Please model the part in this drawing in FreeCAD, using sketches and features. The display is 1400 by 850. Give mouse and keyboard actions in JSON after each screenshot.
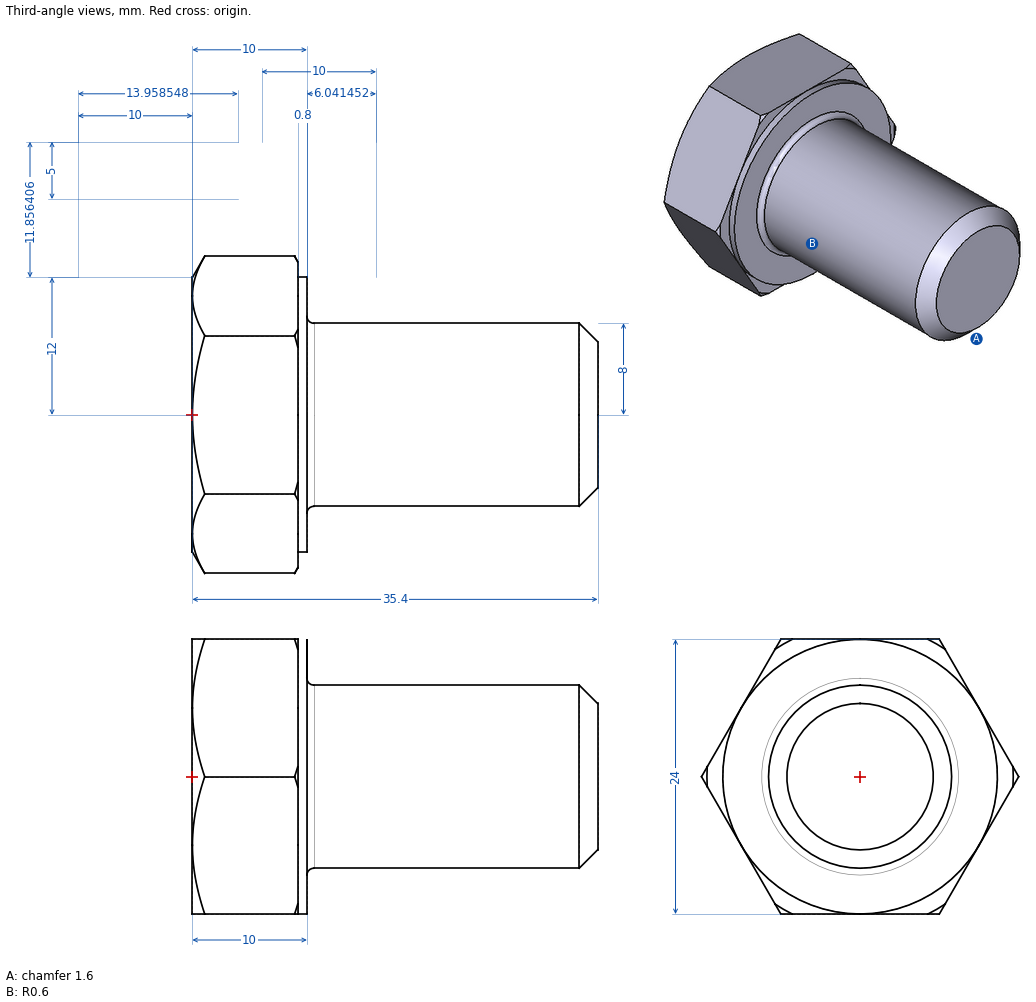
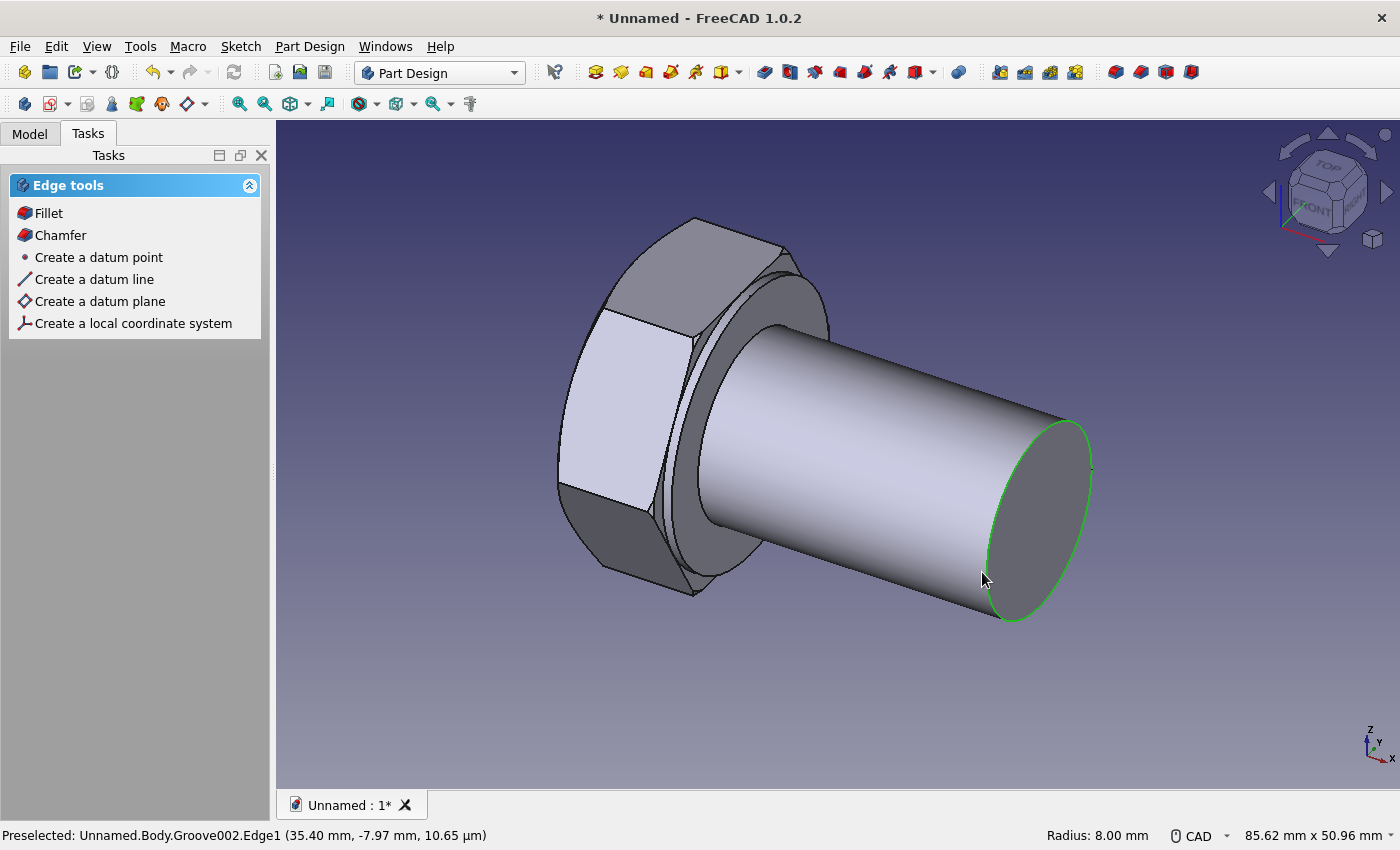
{"action": "left_click", "coordinate": [1141, 72]}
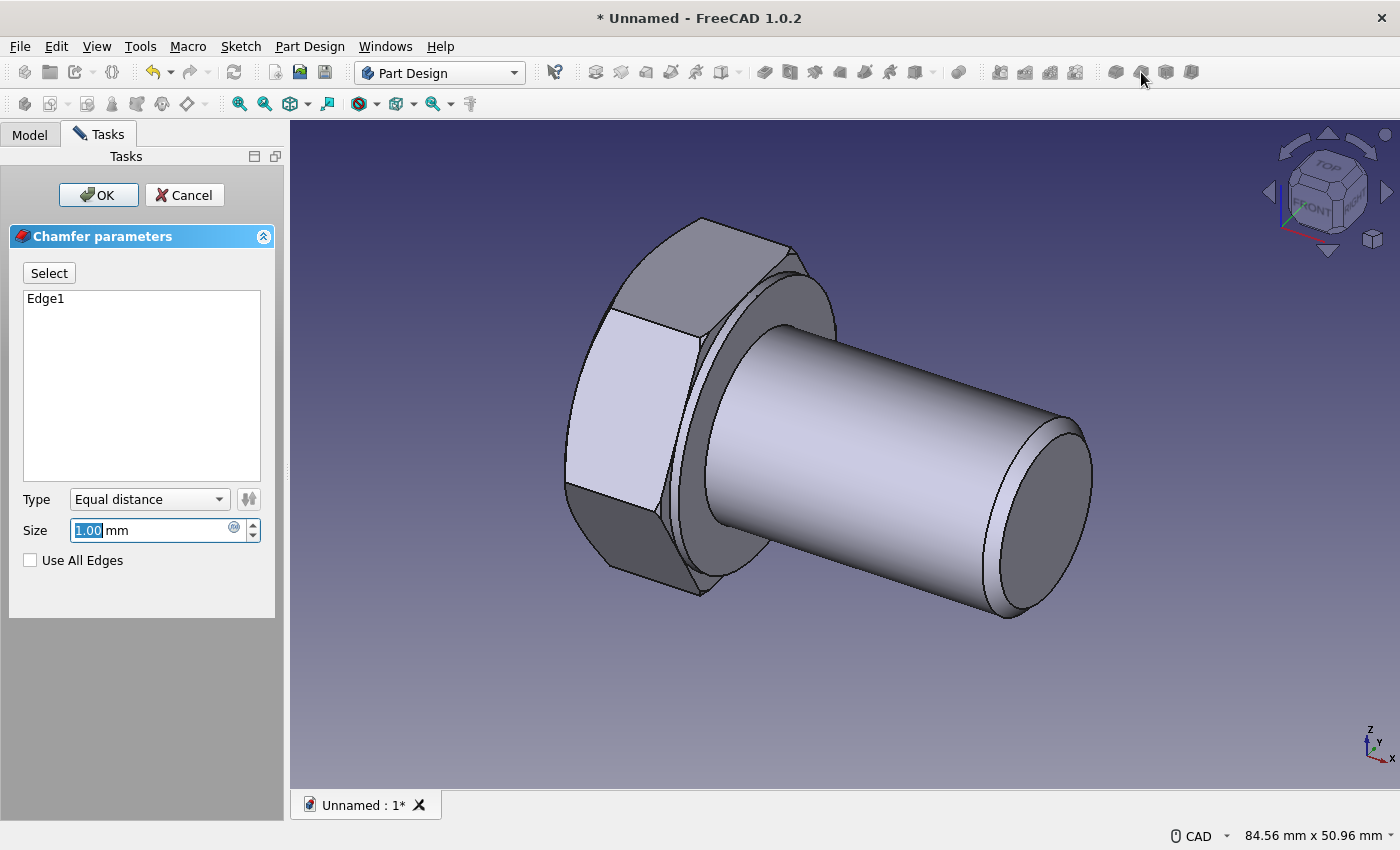
{"action": "type", "text": "1.6"}
{"action": "key", "text": "Tab"}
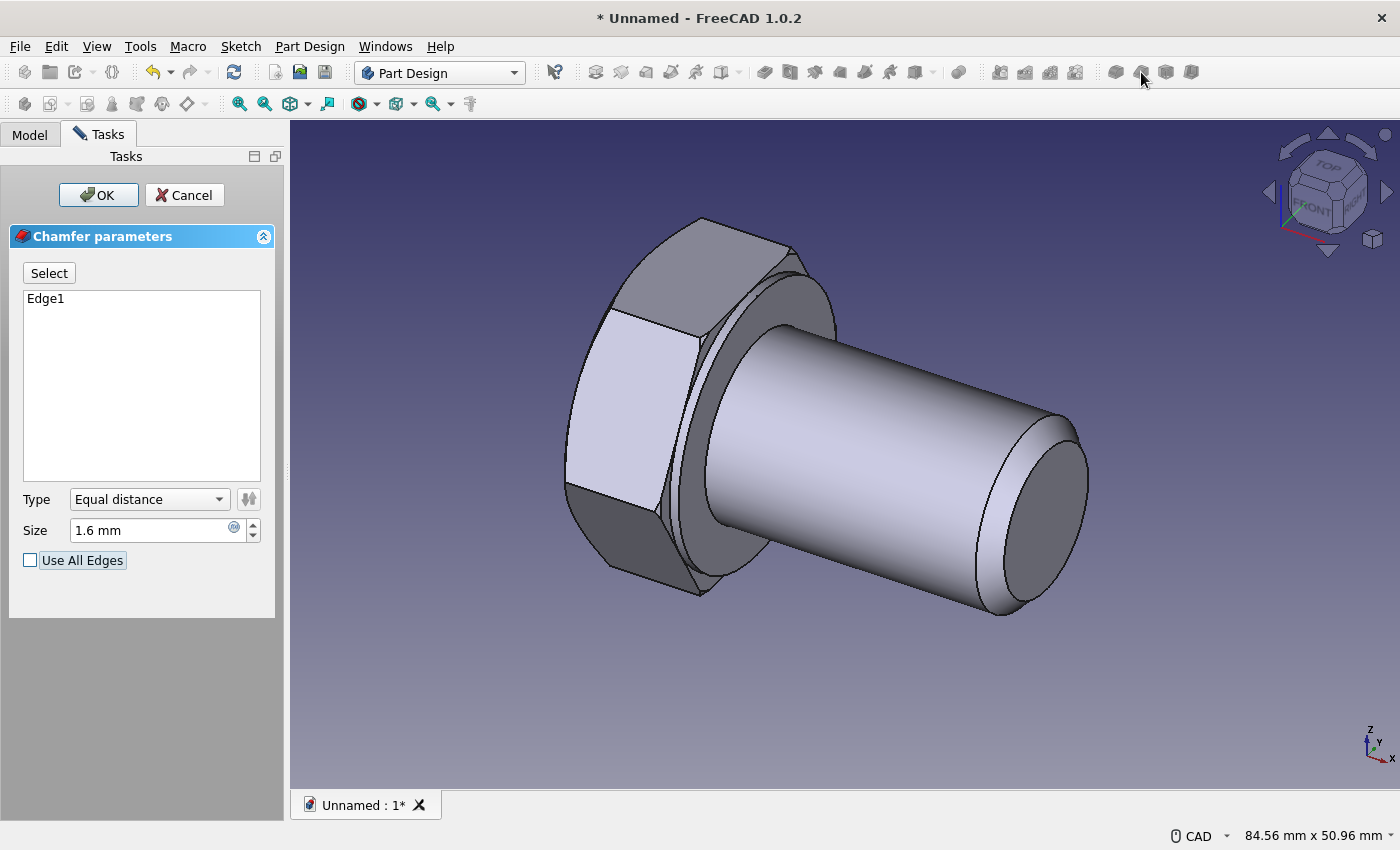
{"action": "left_click", "coordinate": [99, 195]}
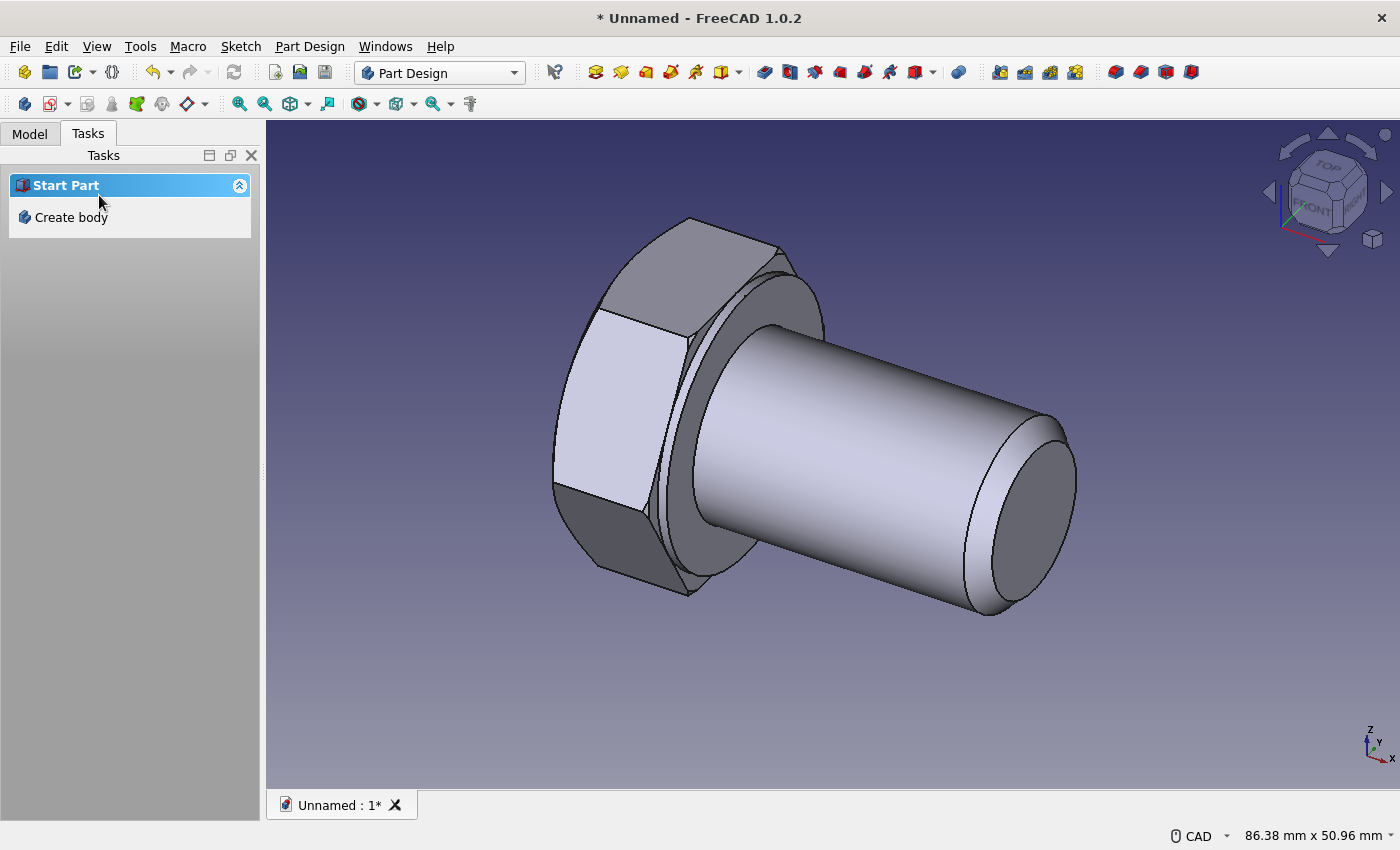
{"action": "key", "text": "0"}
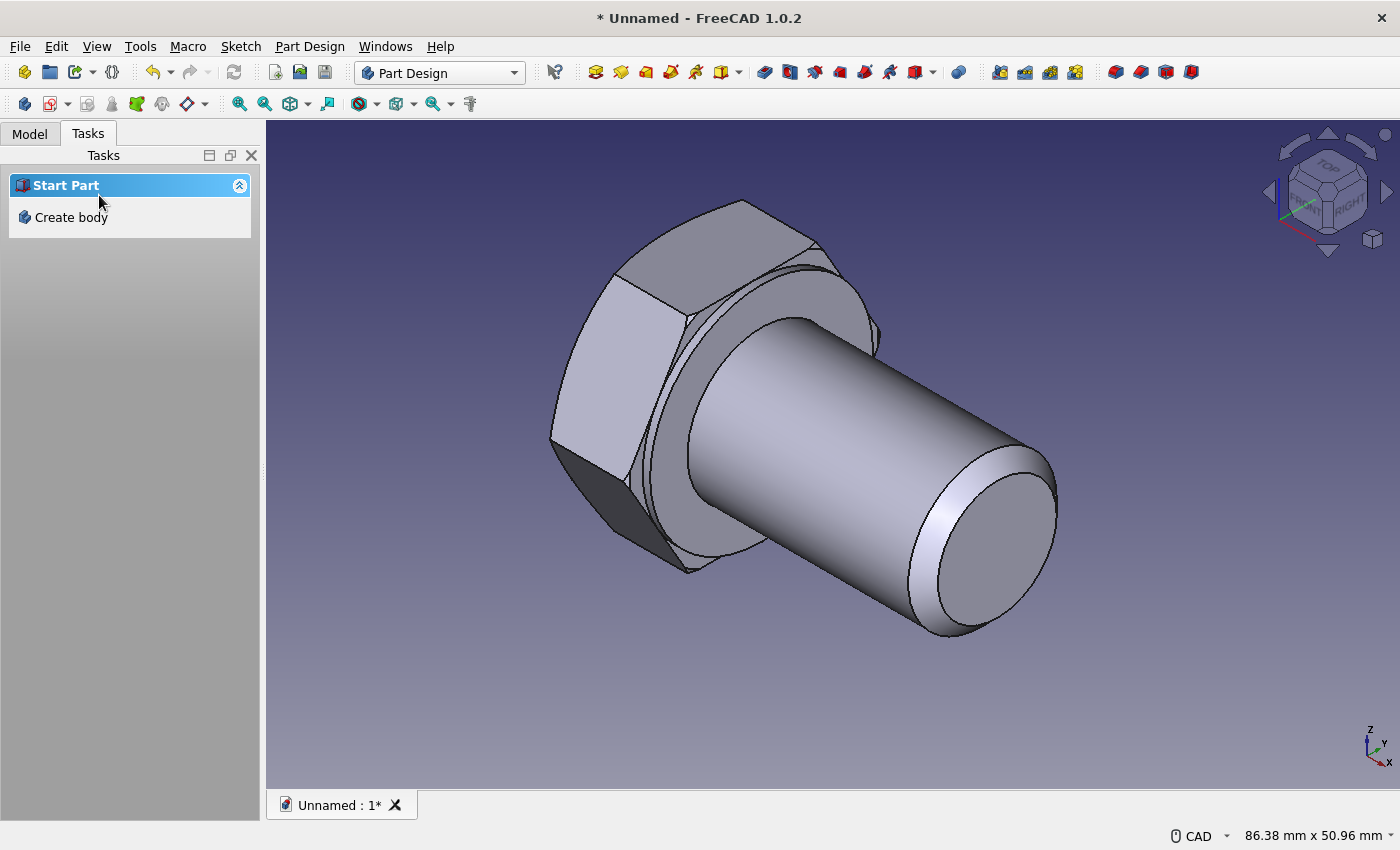
{"action": "key", "text": "2"}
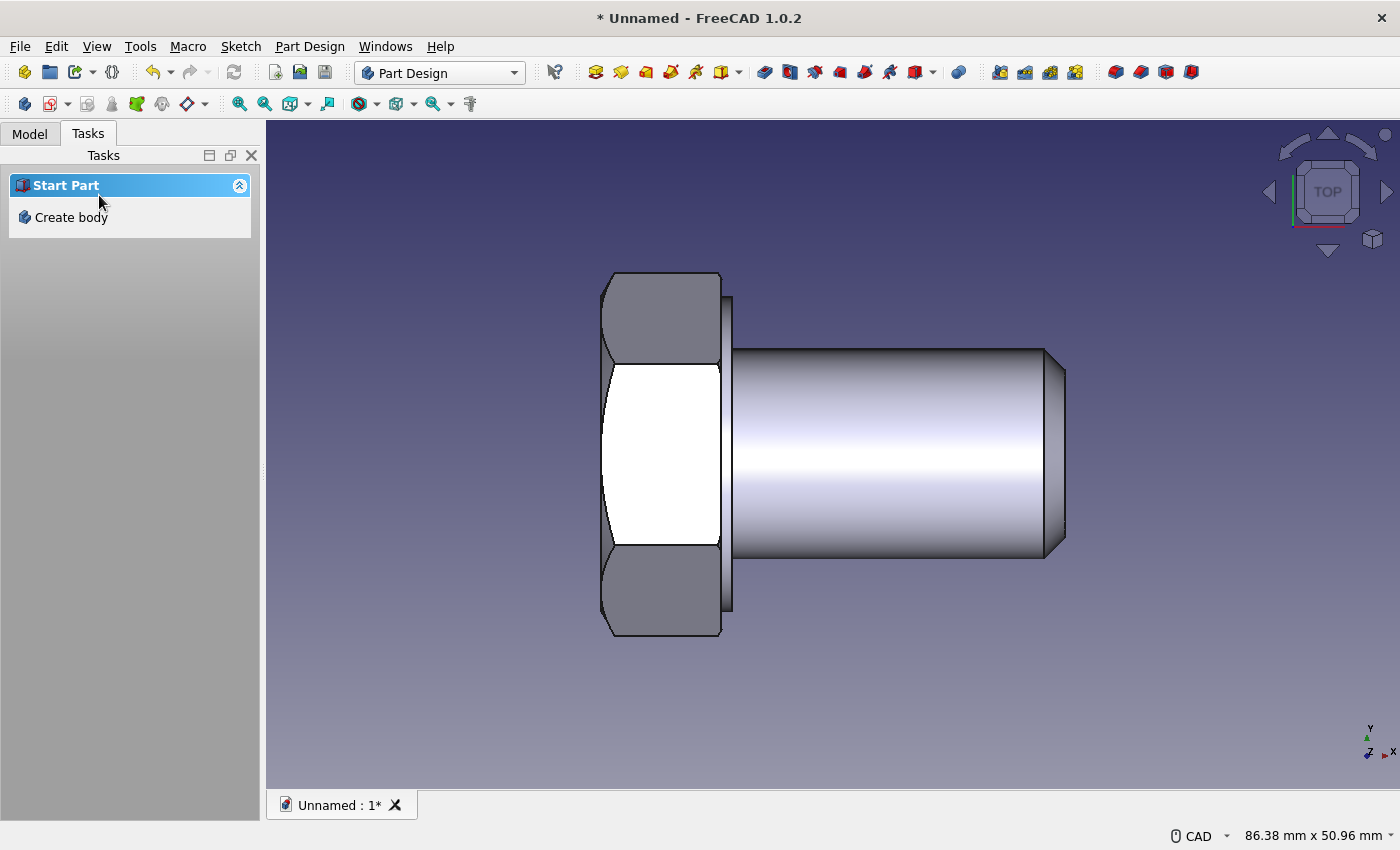
{"action": "key", "text": "1"}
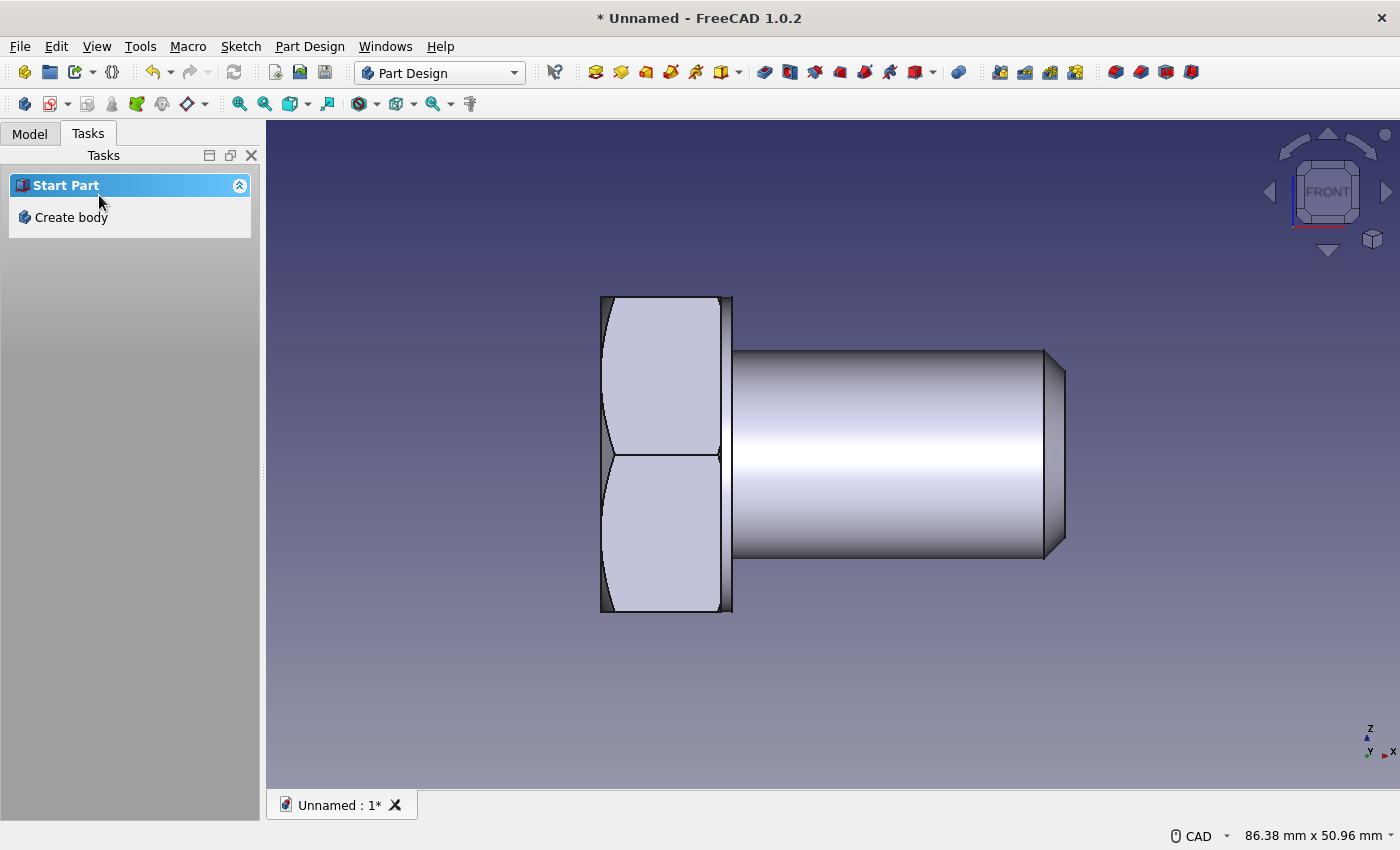
{"action": "key", "text": "3"}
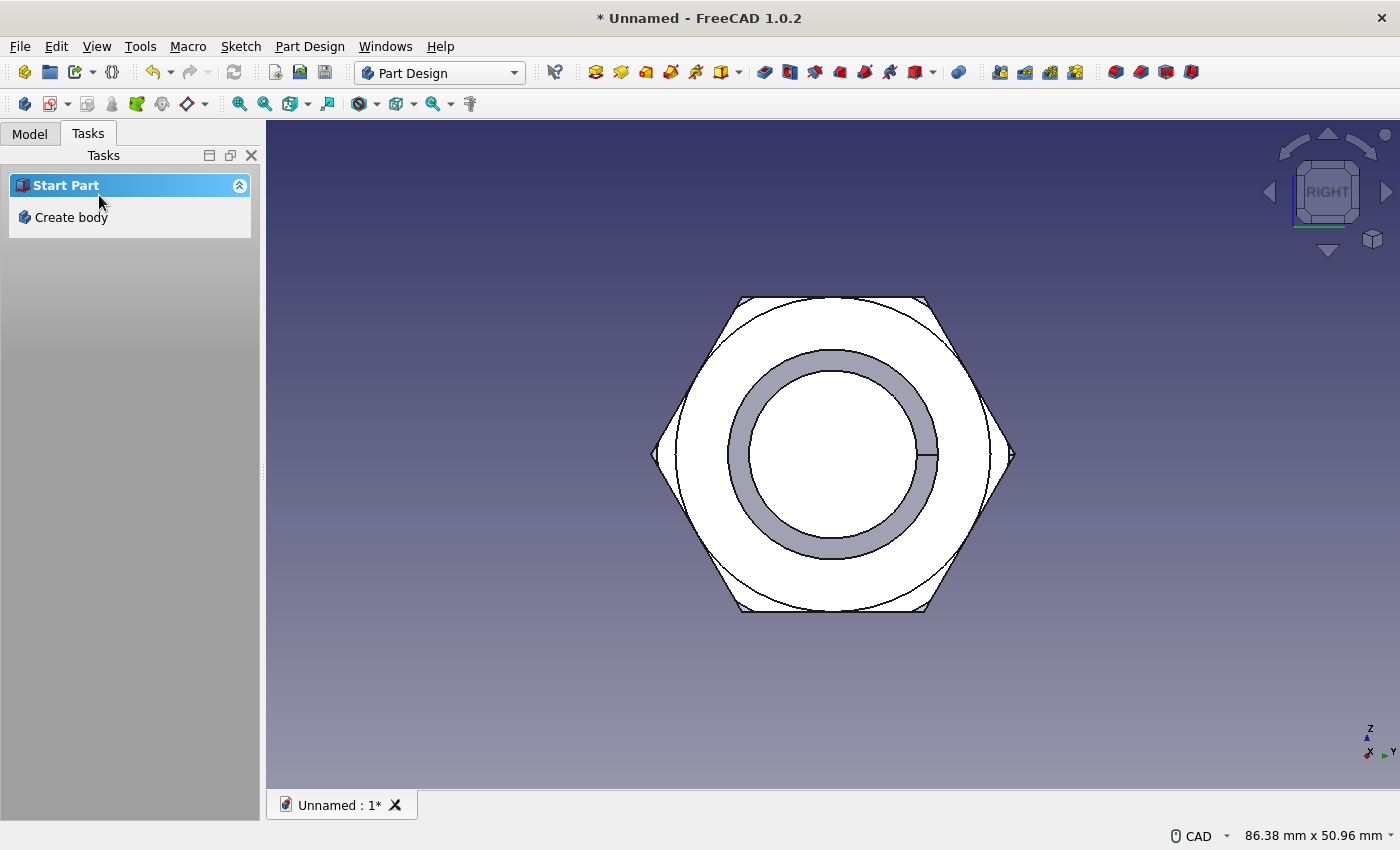
{"action": "key", "text": "5"}